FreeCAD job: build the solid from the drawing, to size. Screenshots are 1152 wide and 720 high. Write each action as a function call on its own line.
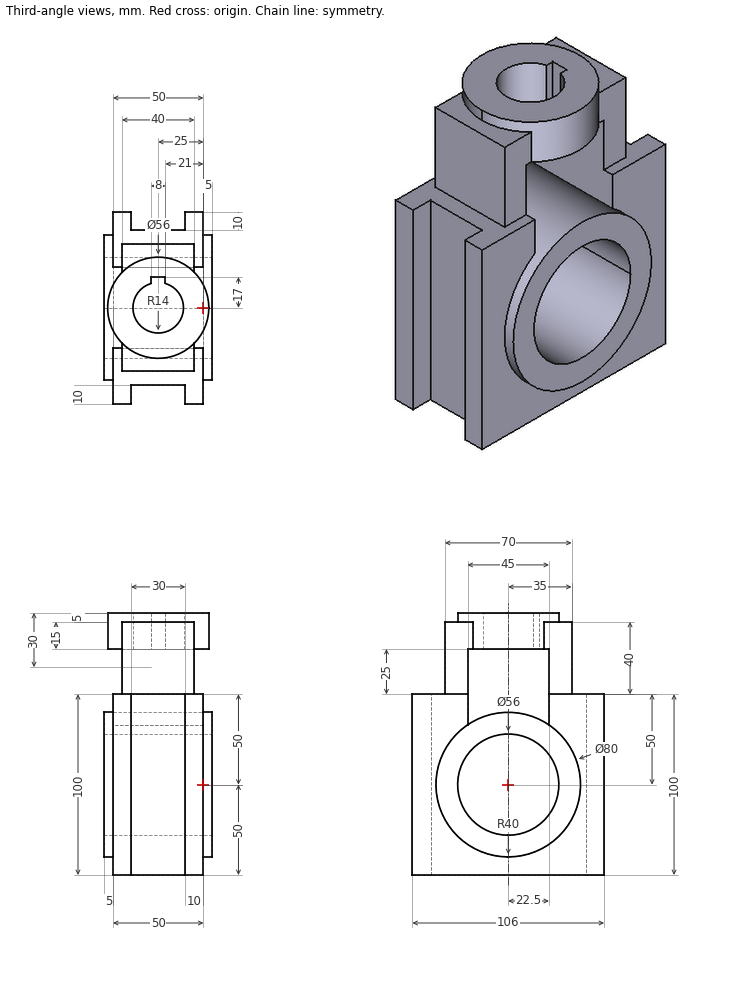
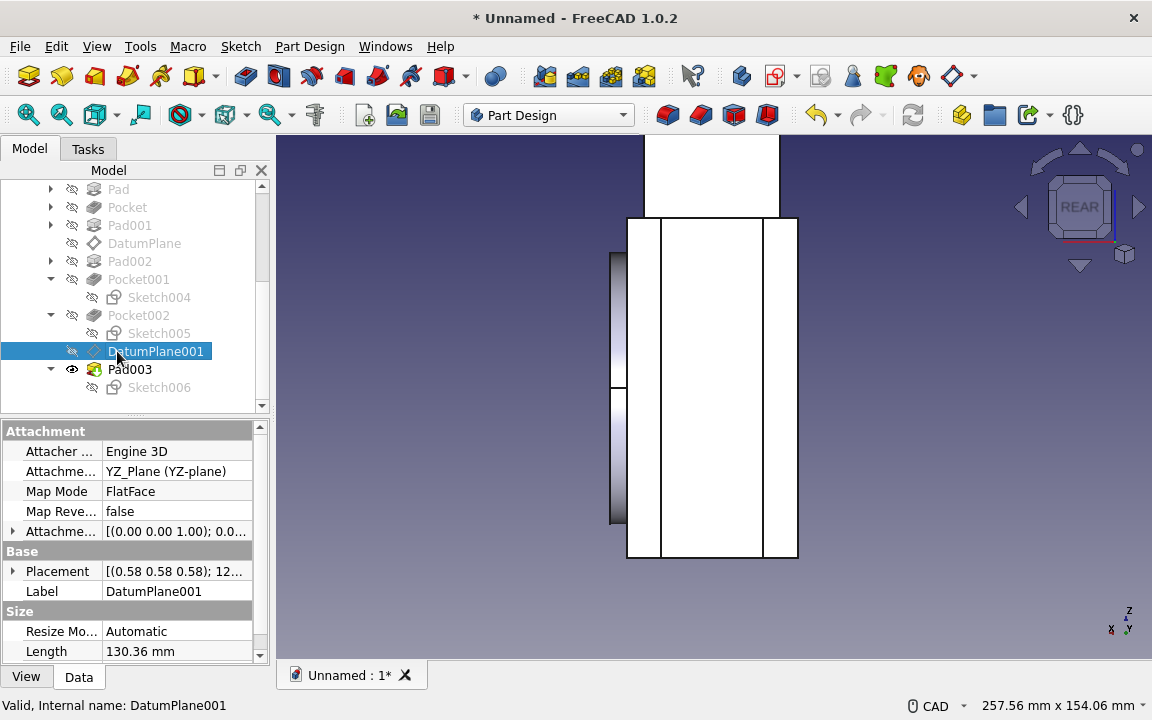
key(v)
key(f)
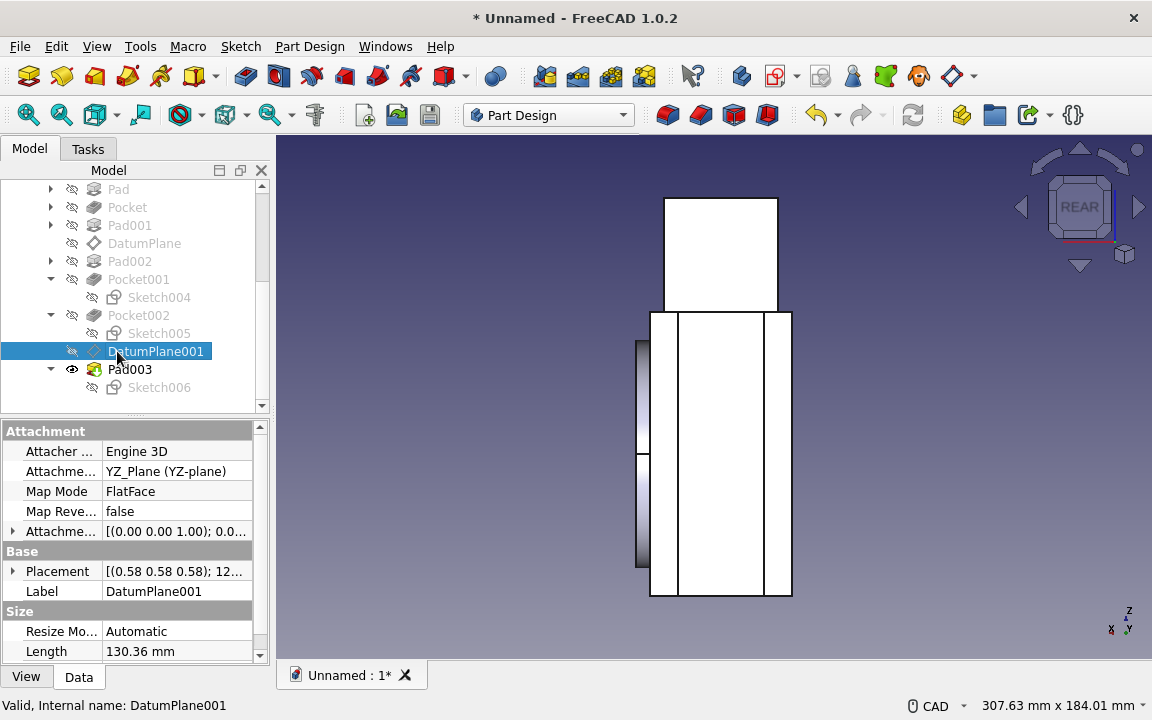
key(0)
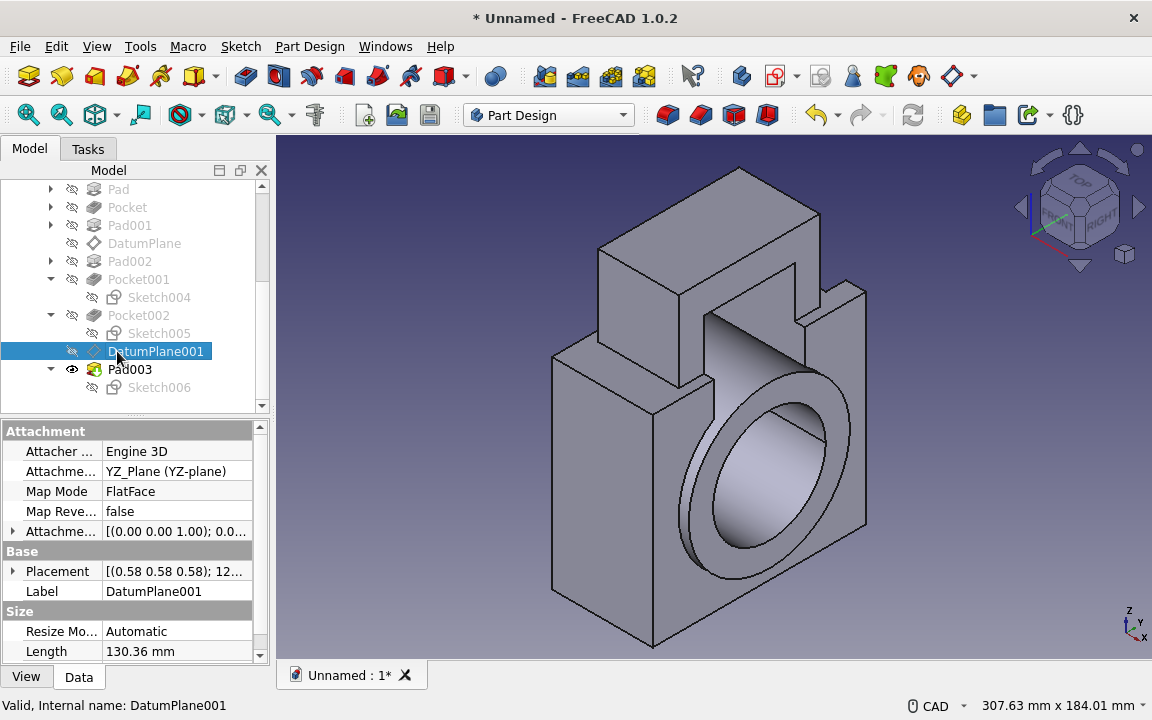
click(729, 219)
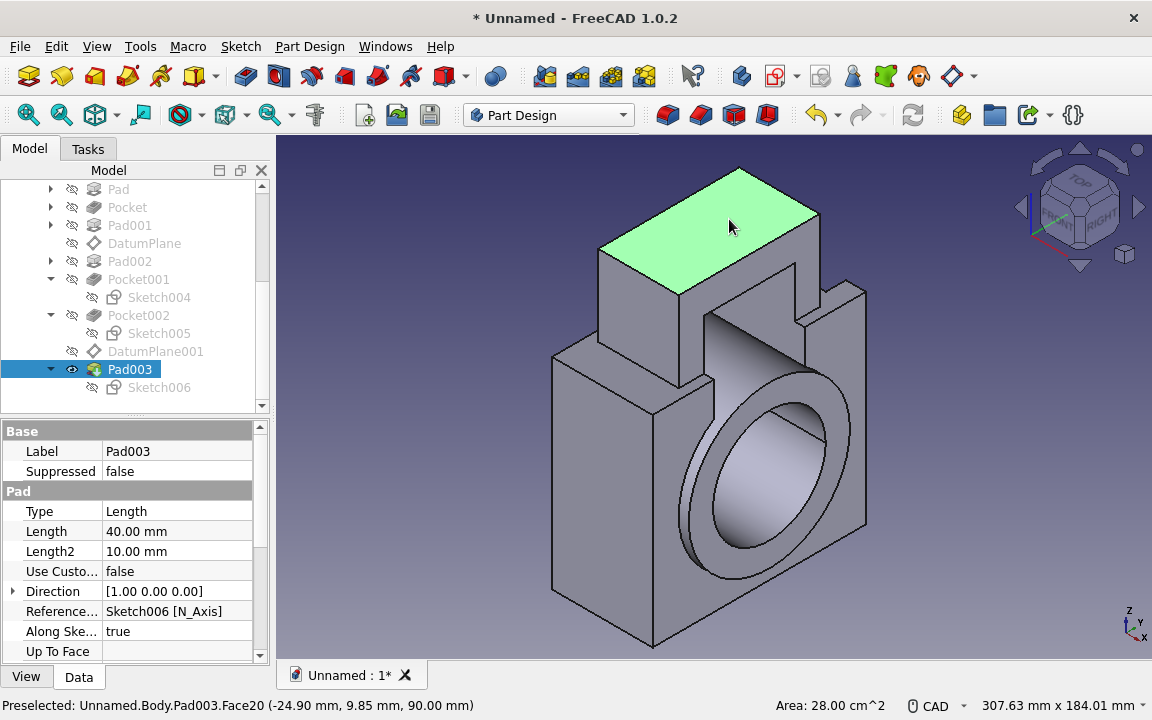
click(774, 76)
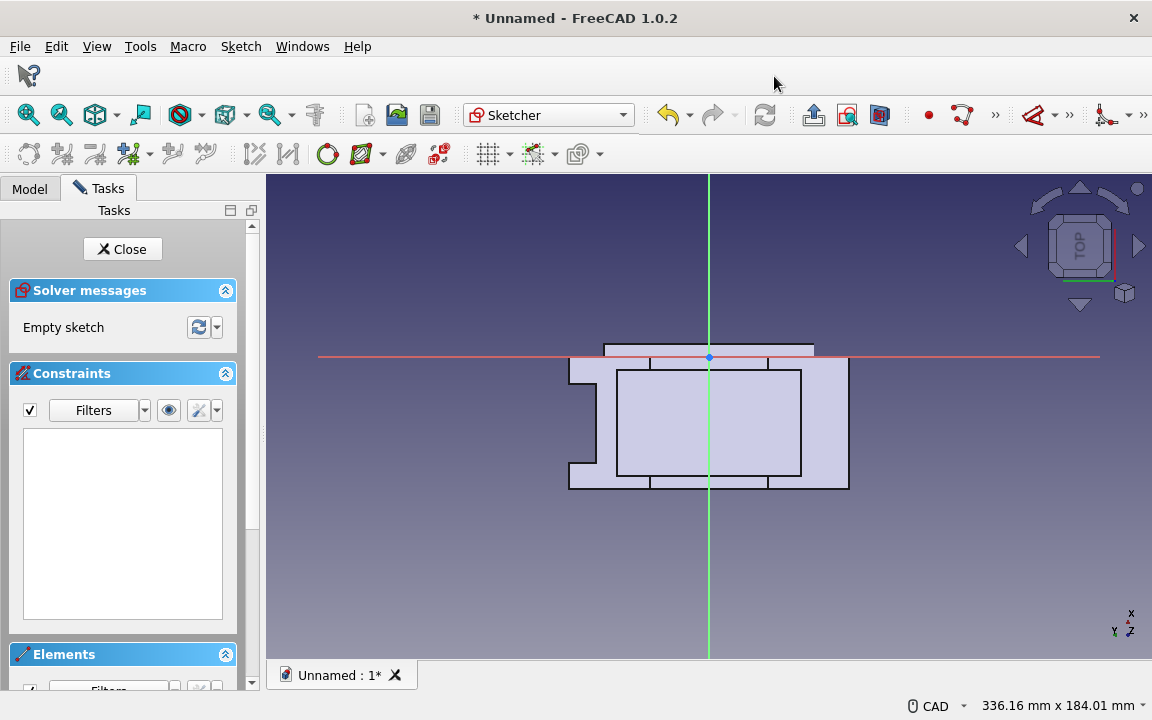
scroll(765, 428, up, 4)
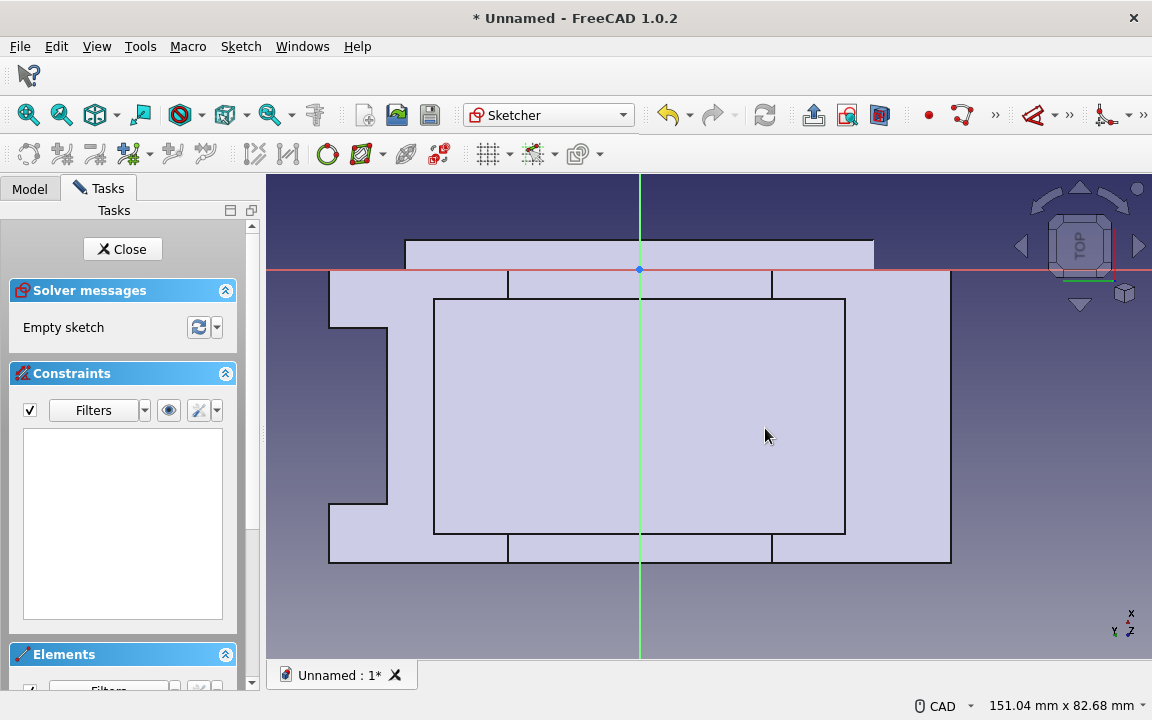
key(g)
key(c)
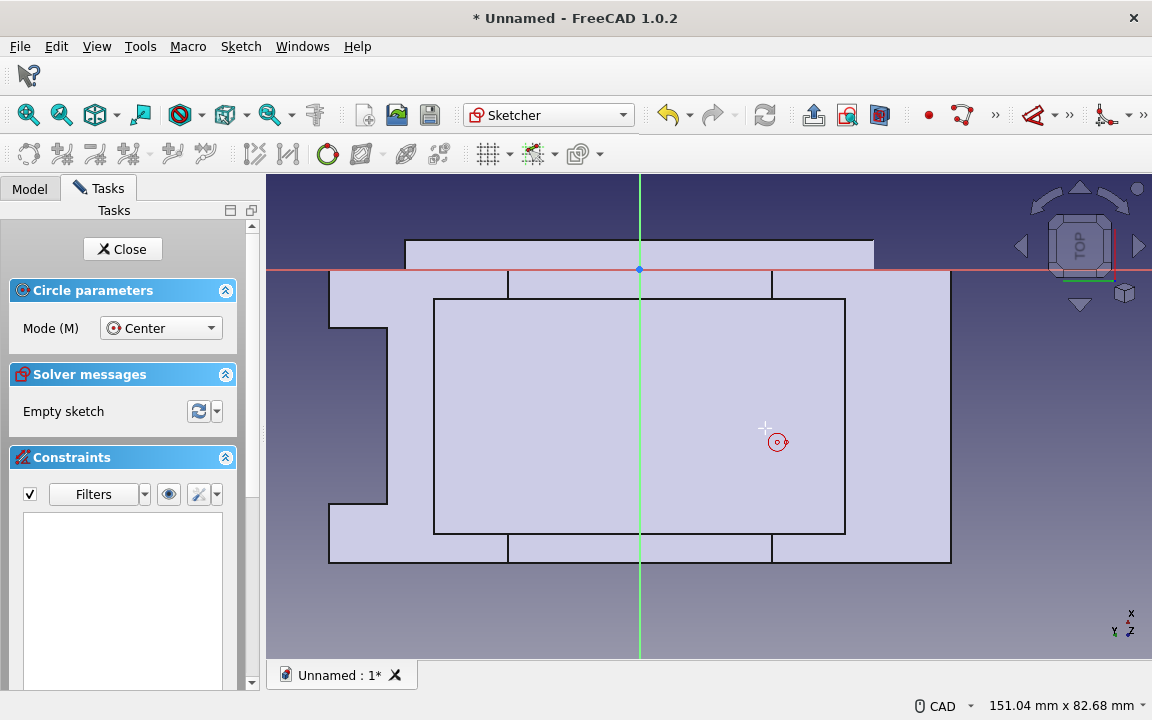
click(640, 416)
move(756, 300)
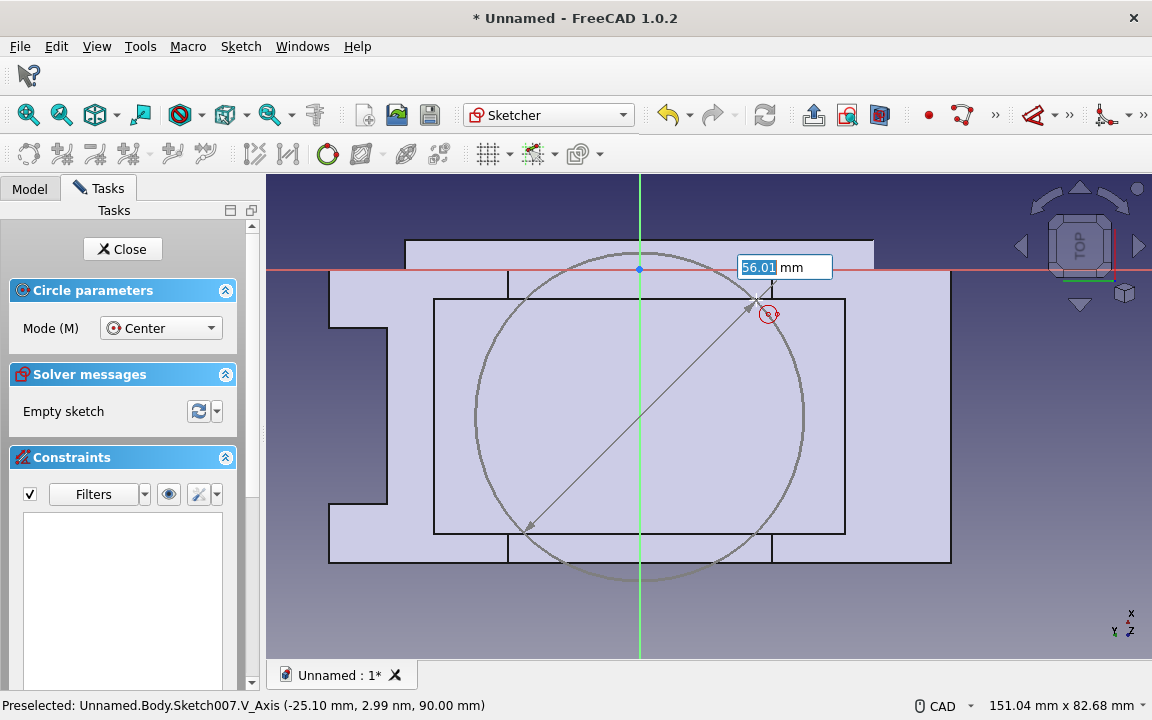
text(56)
key(Return)
key(Escape)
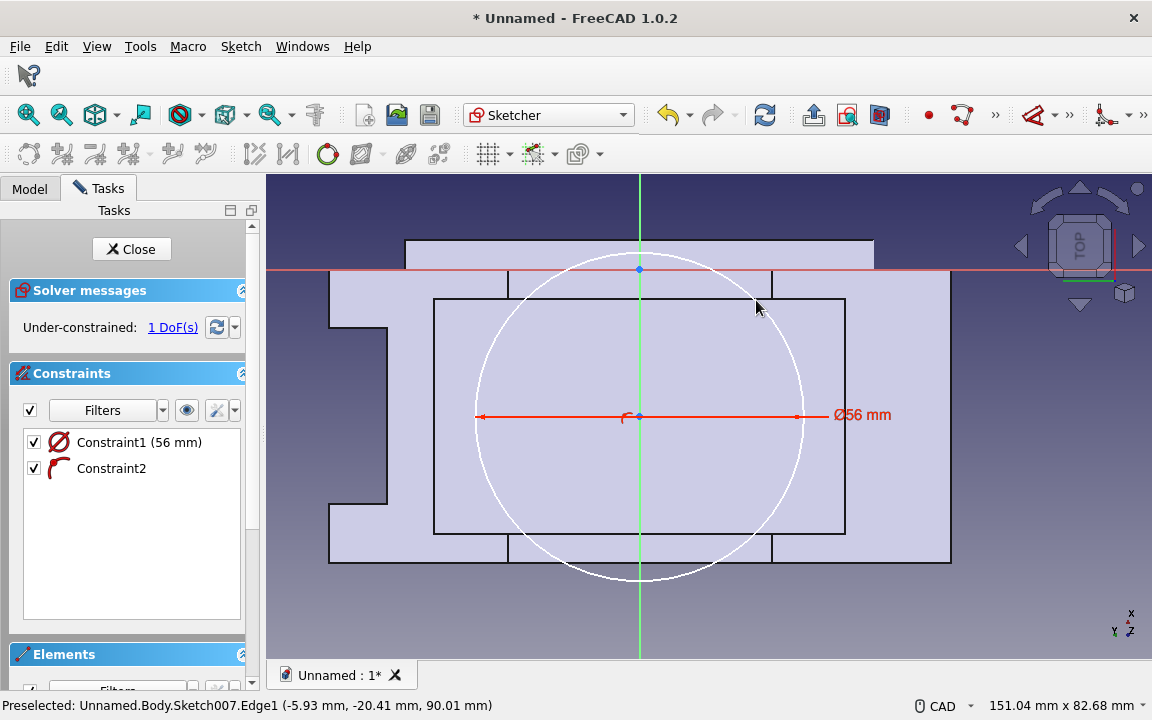
key(d)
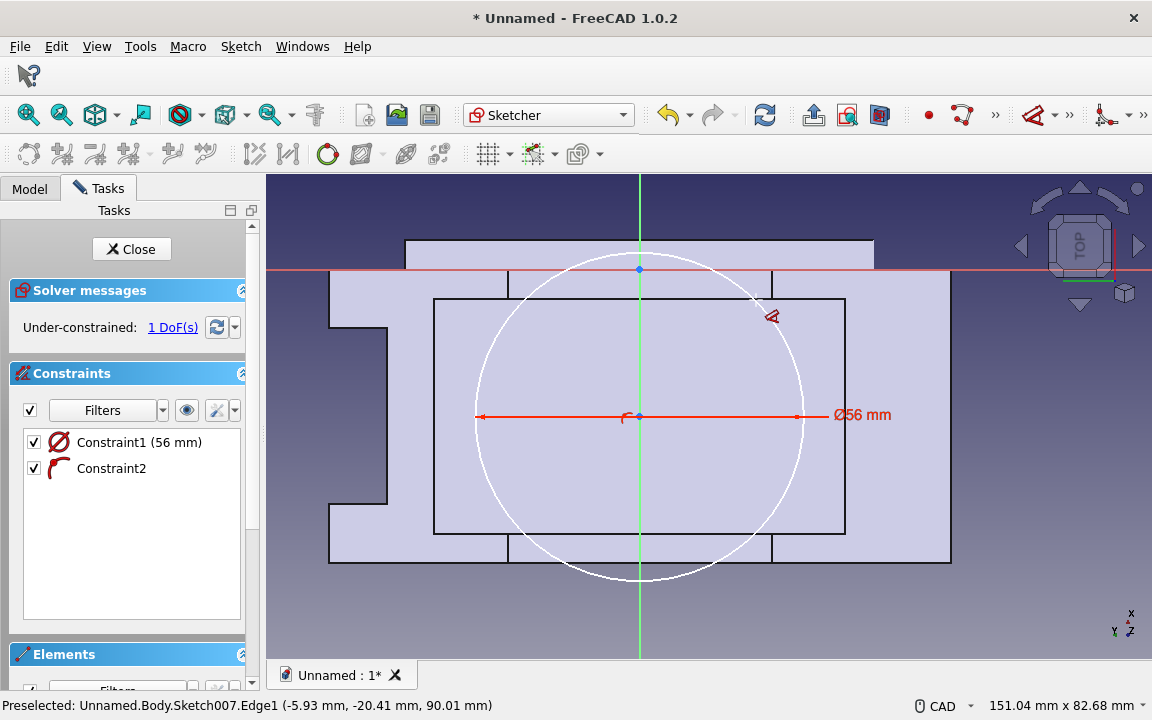
click(640, 417)
click(674, 343)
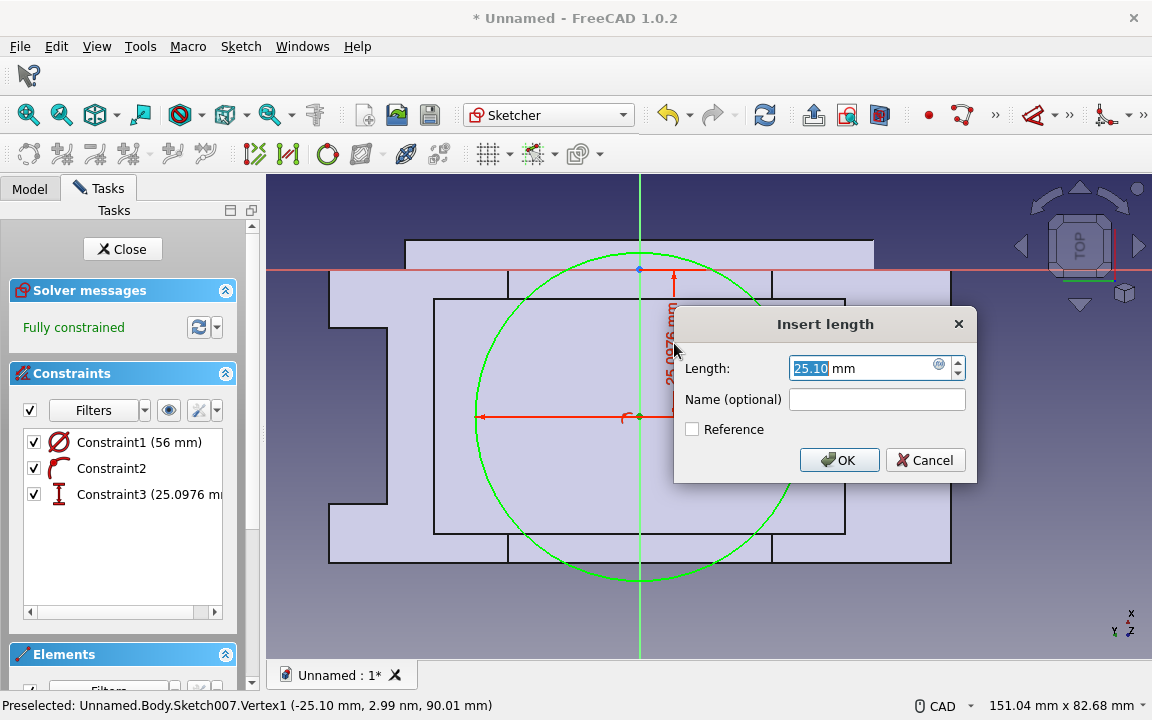
text(25)
key(Return)
key(Escape)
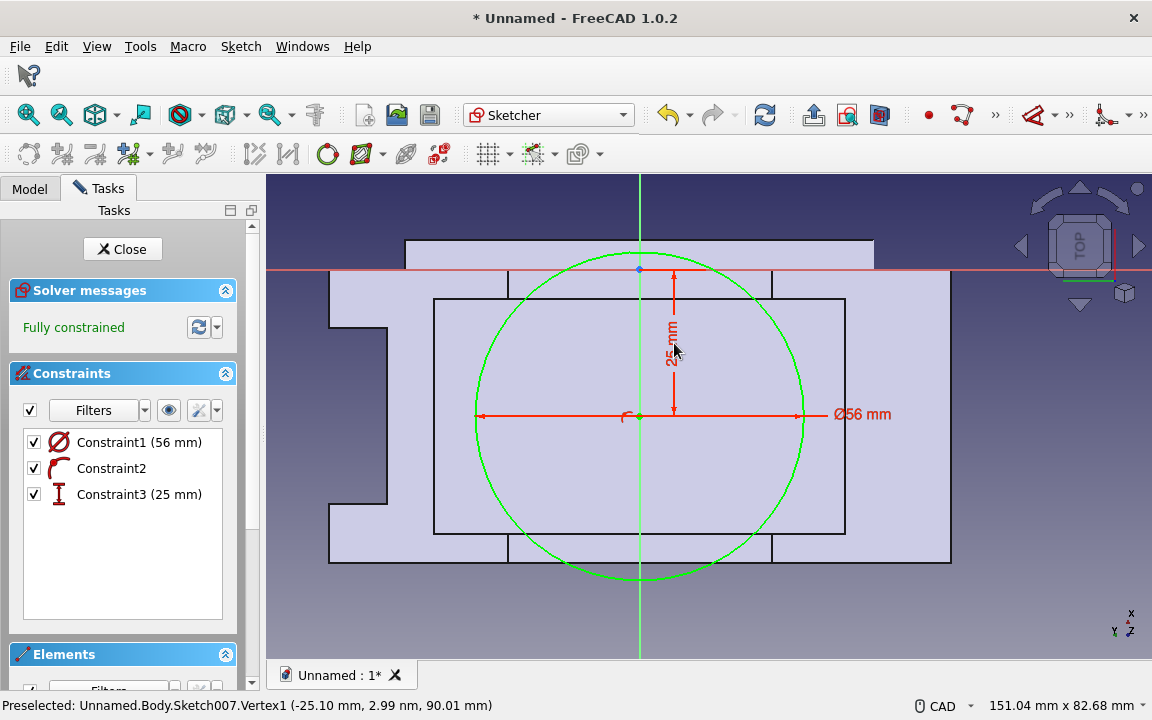
click(123, 249)